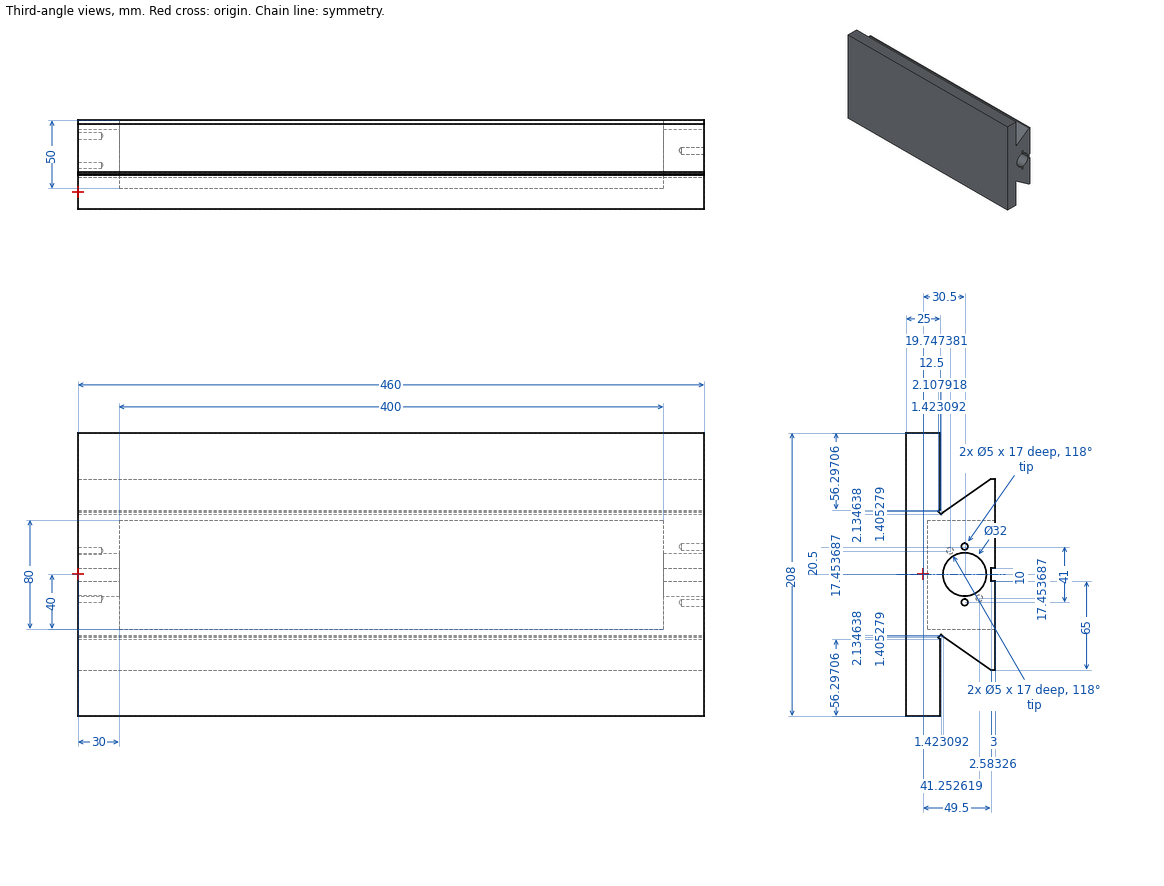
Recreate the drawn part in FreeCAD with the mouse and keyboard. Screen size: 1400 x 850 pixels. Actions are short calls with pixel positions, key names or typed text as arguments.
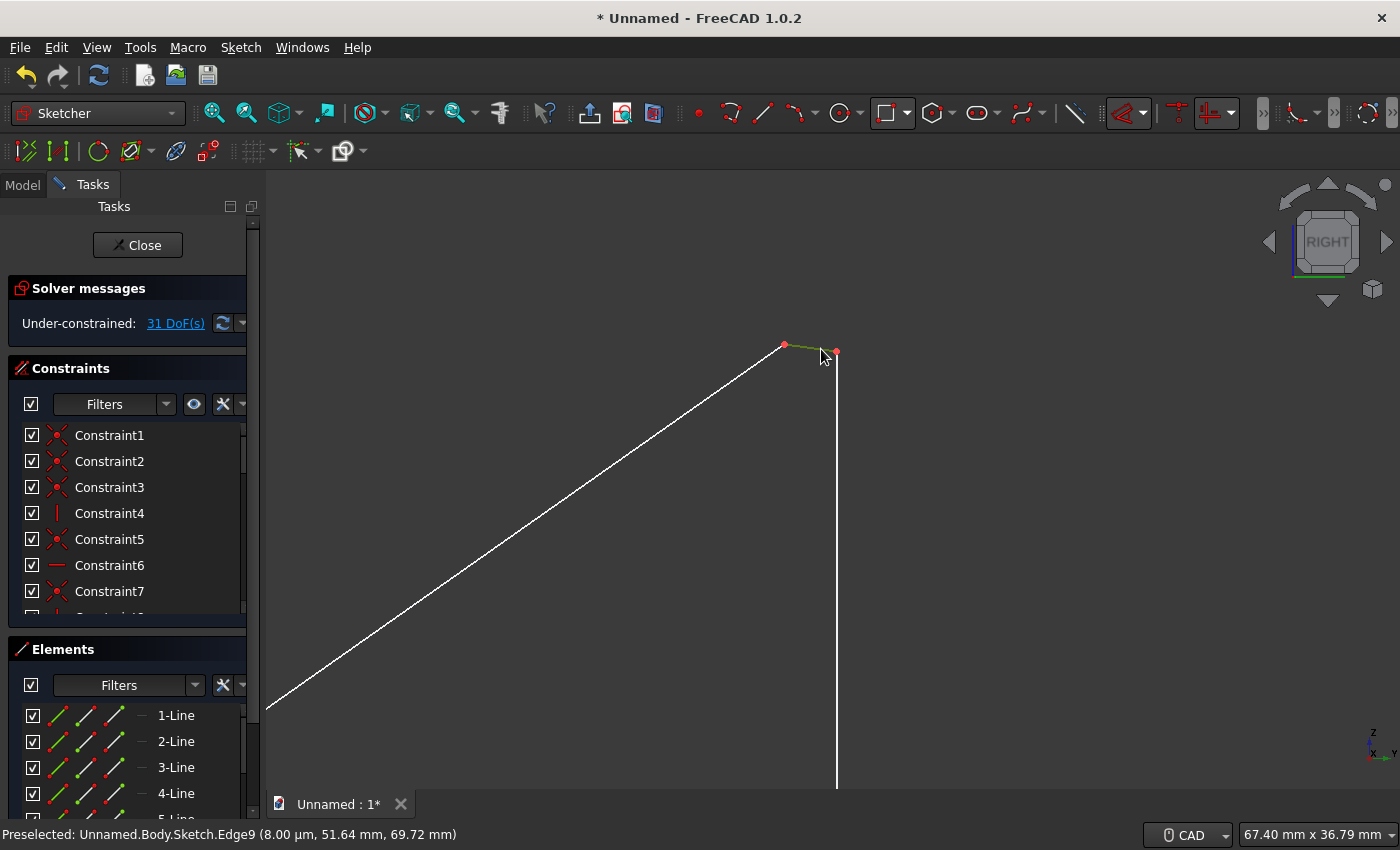
click(1234, 114)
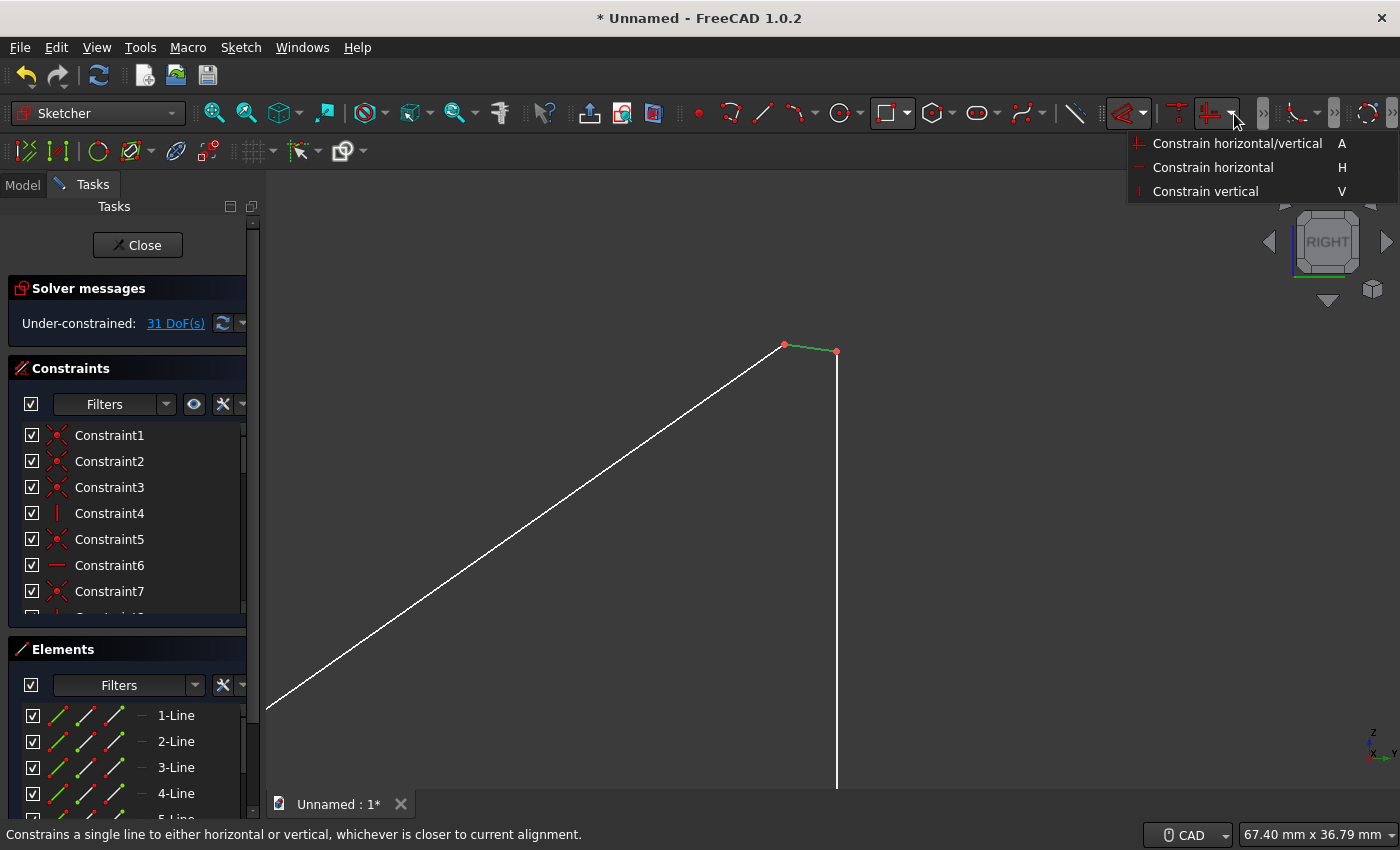
click(1263, 167)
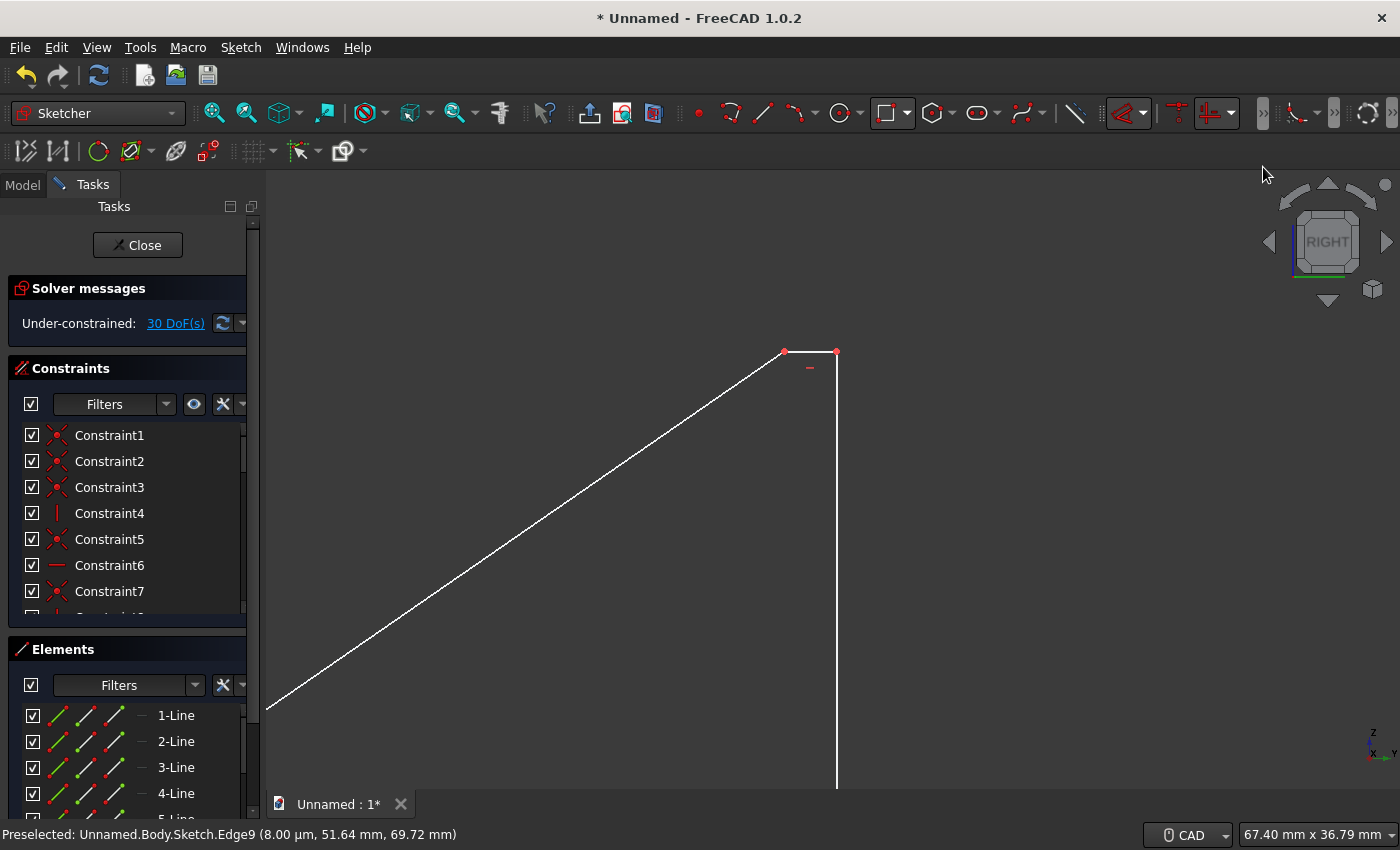
scroll(824, 350, down, 11)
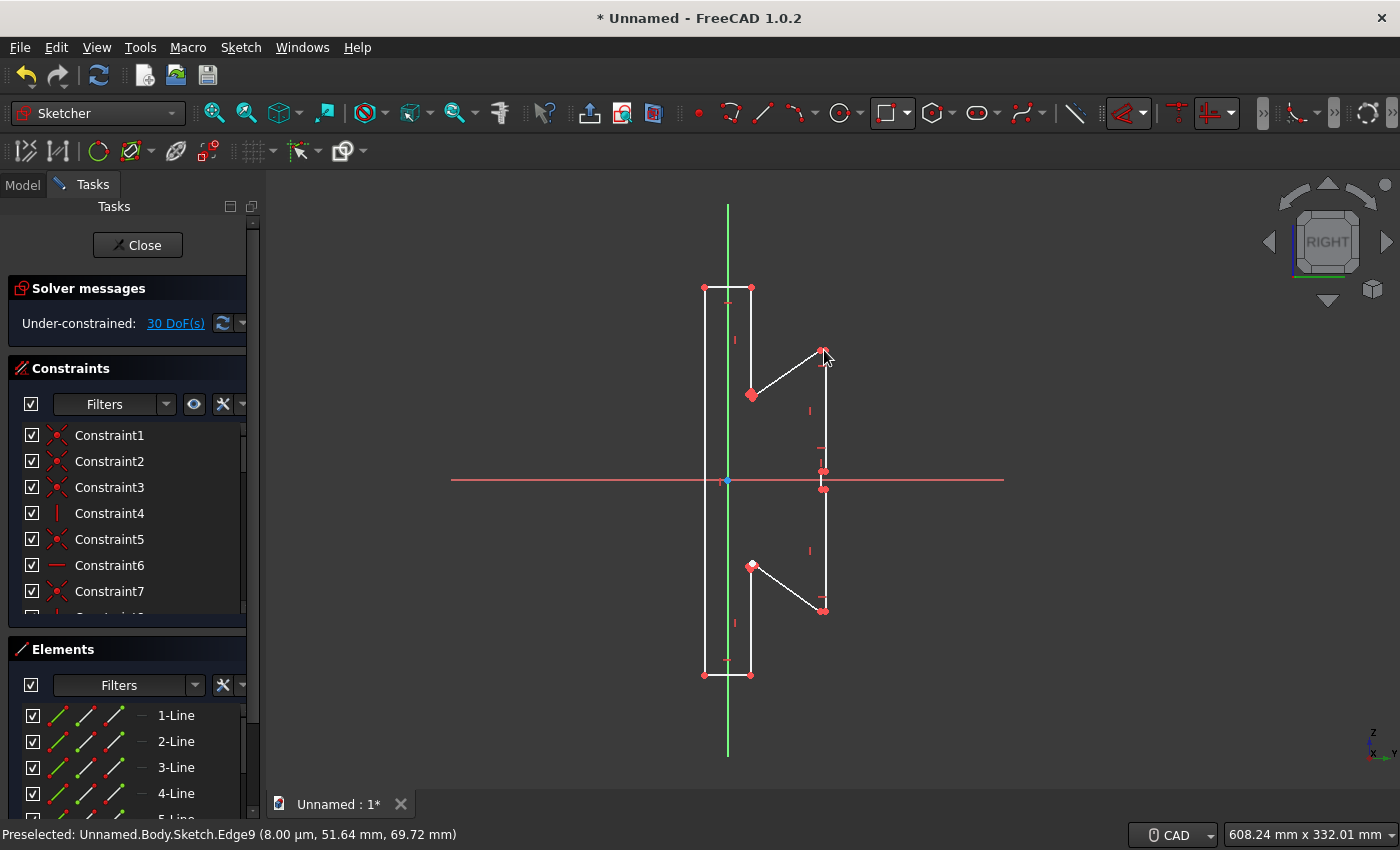
scroll(826, 490, up, 5)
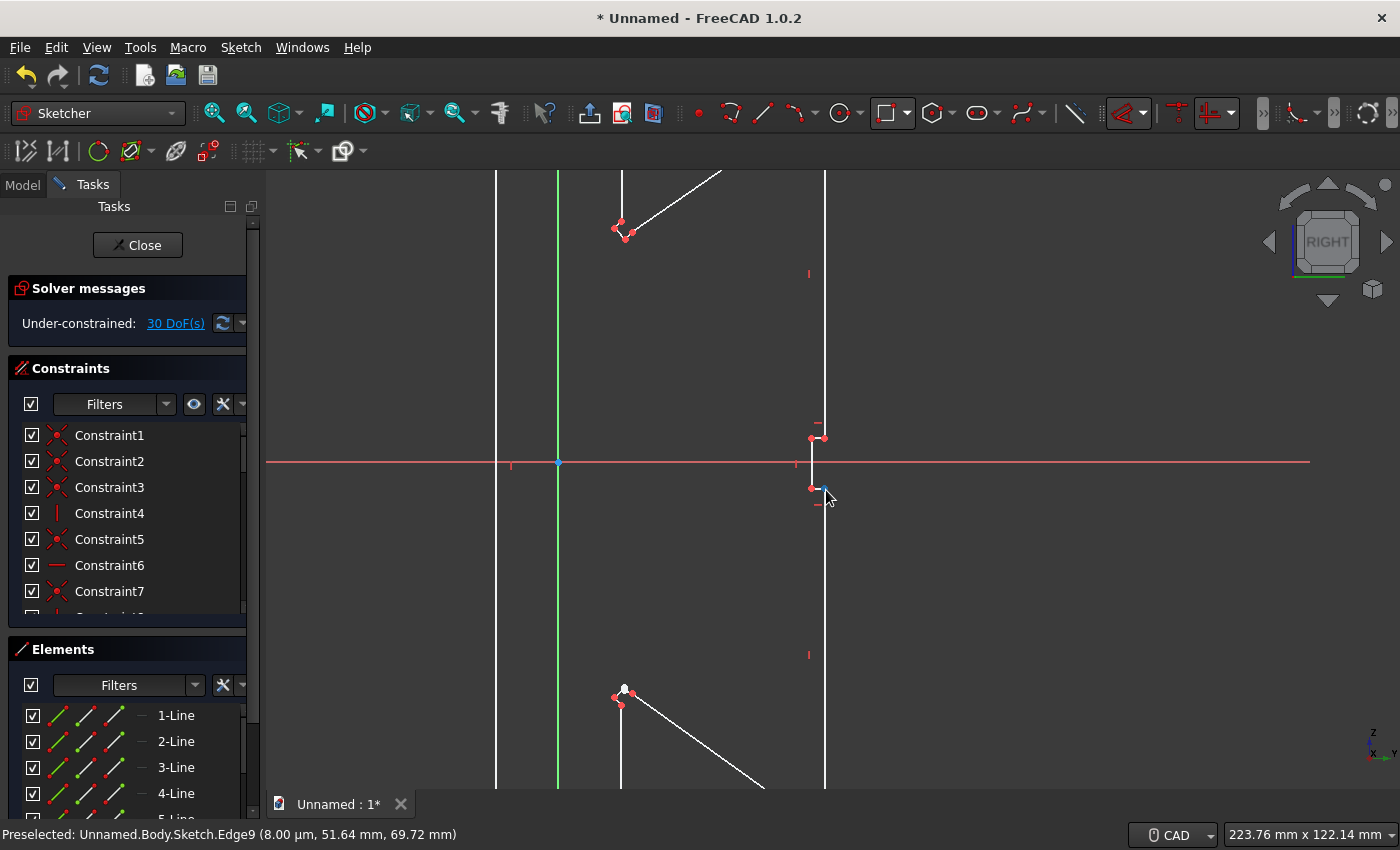
click(825, 489)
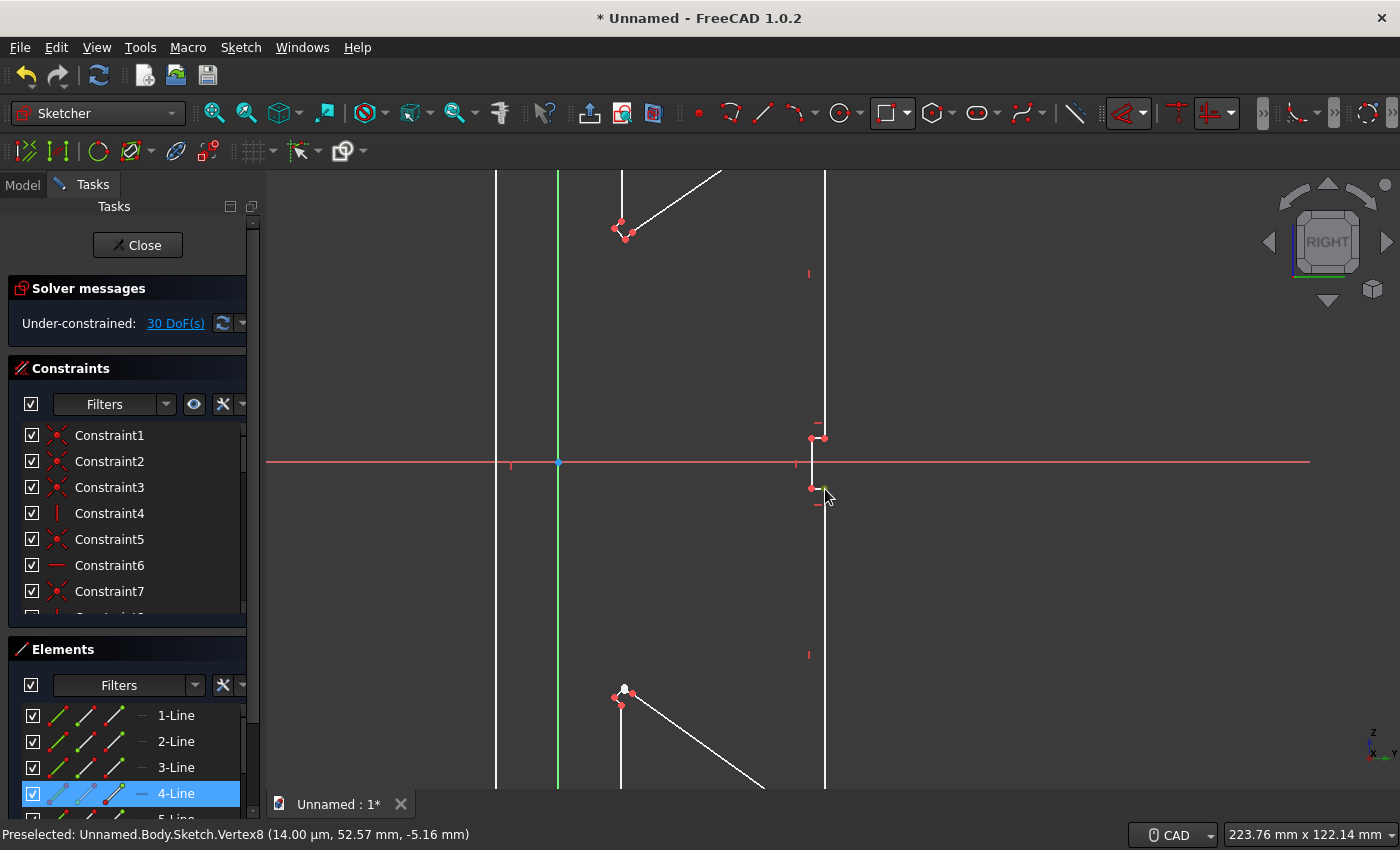
click(825, 438)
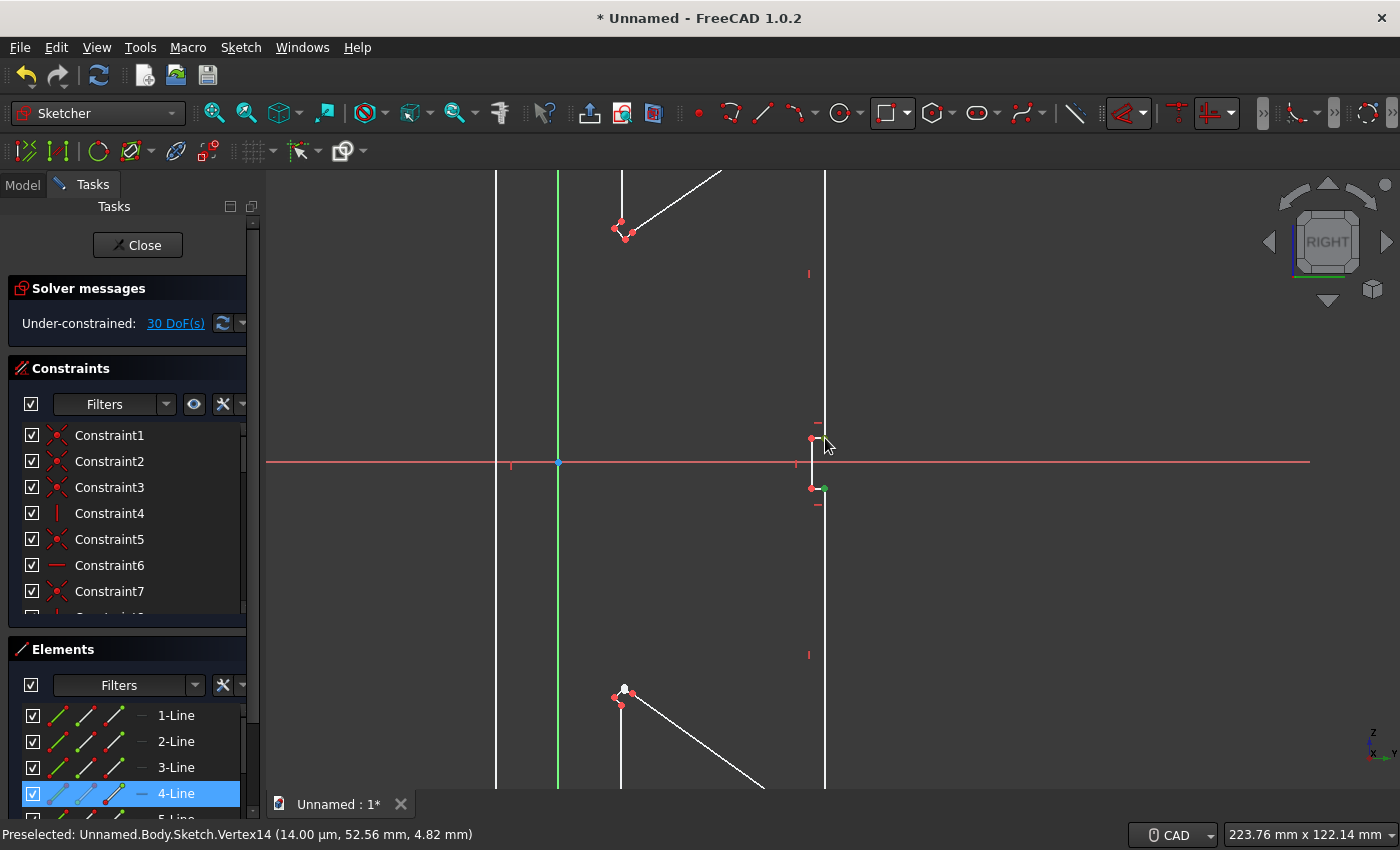
click(361, 462)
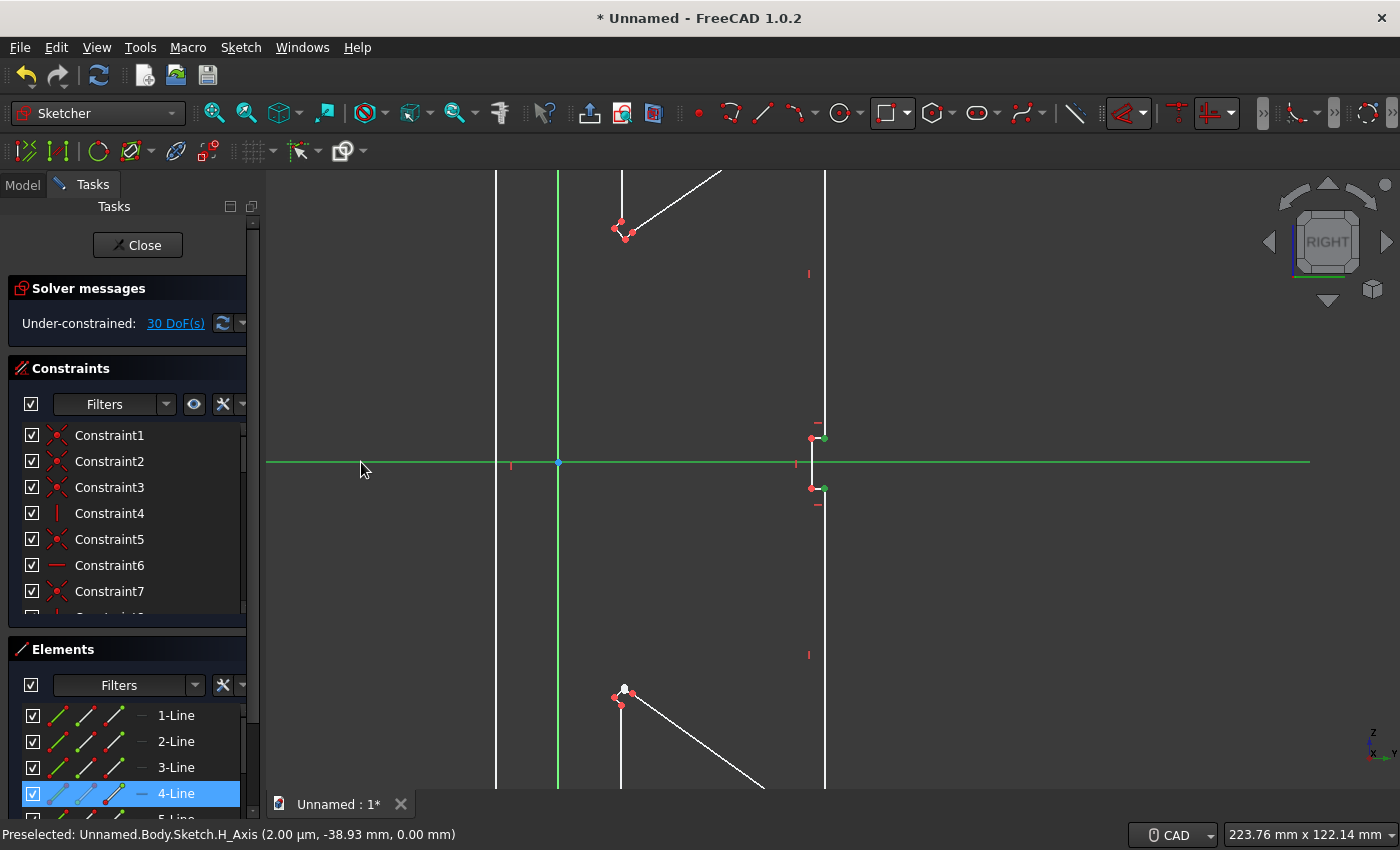
key(s)